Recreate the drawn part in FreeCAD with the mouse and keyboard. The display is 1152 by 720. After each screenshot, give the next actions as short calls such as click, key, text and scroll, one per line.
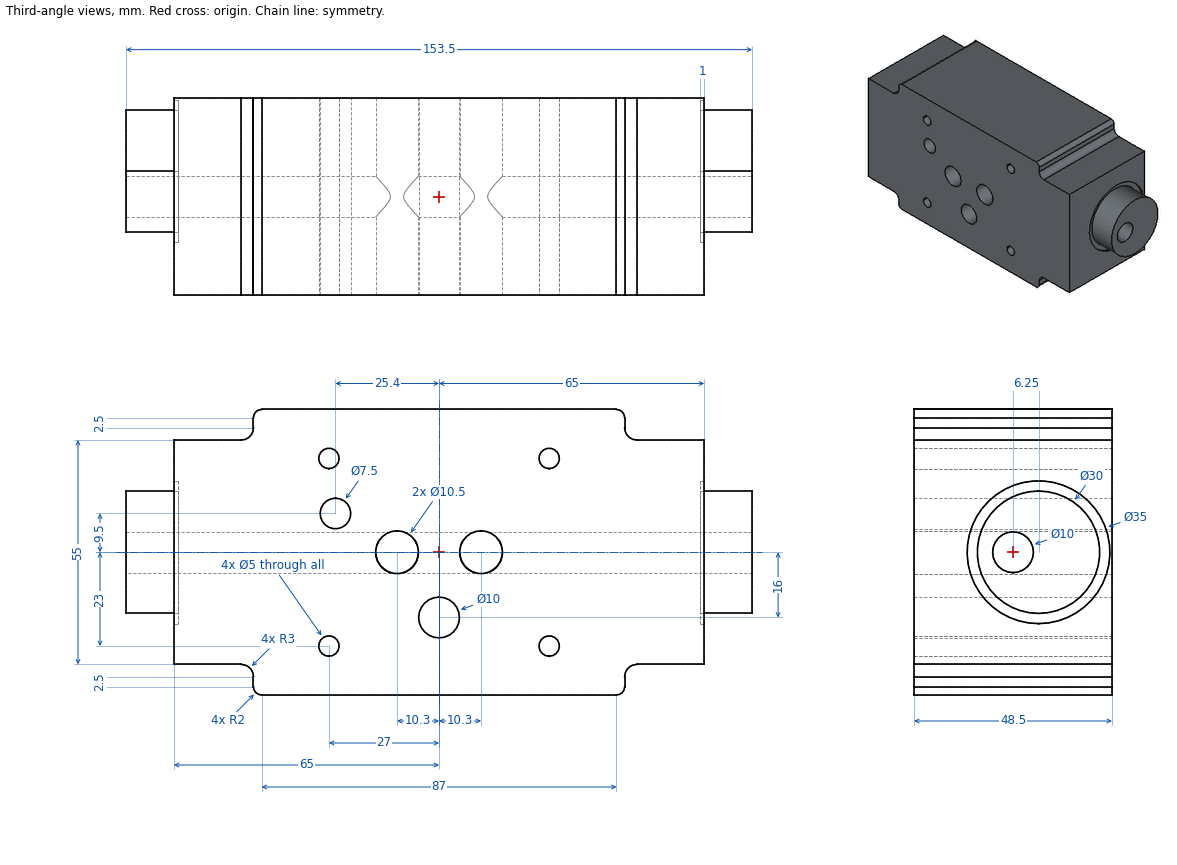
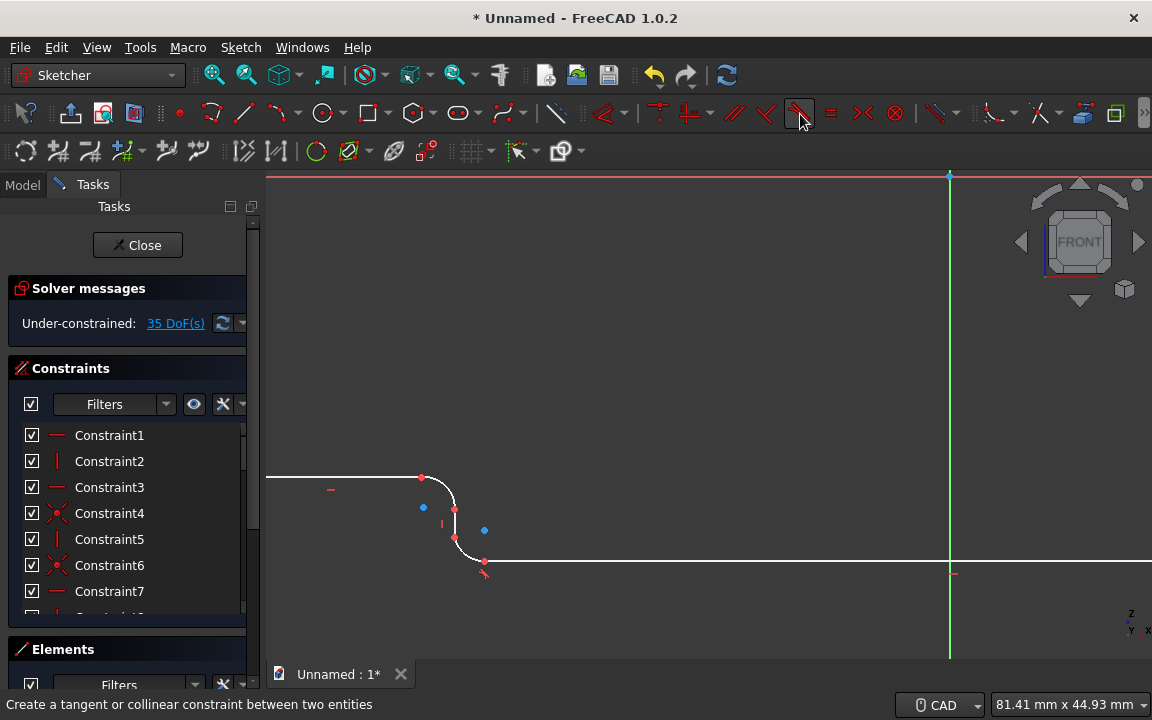
click(766, 561)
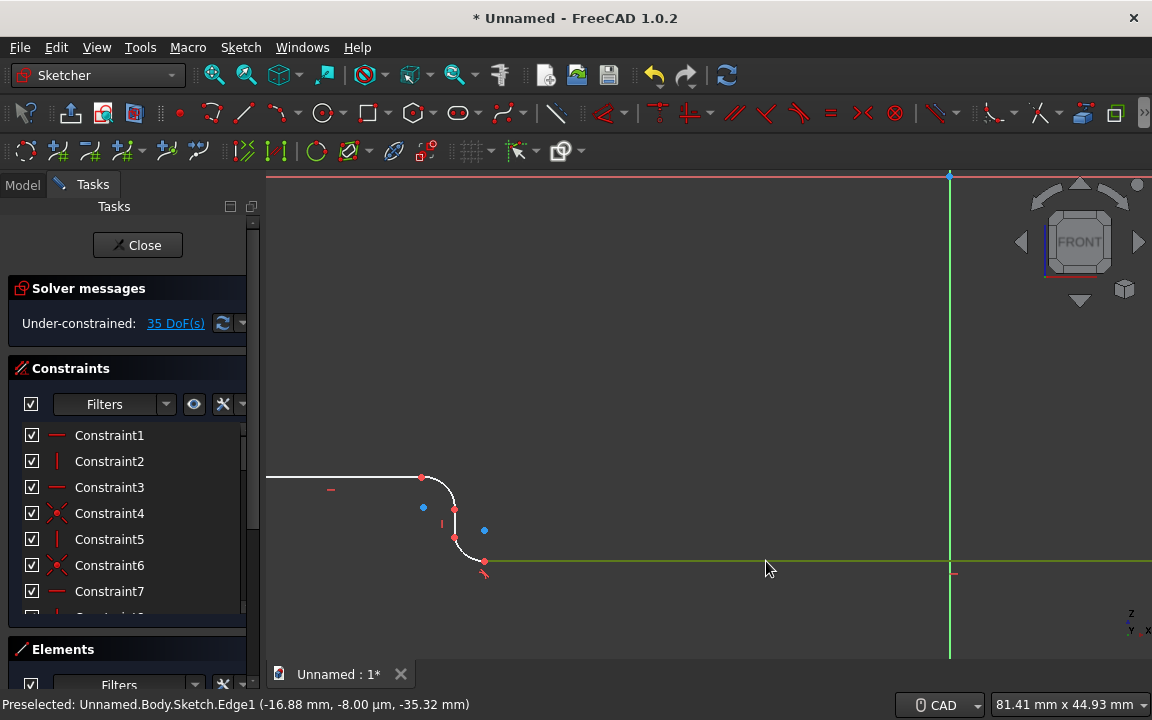
scroll(461, 553, down, 5)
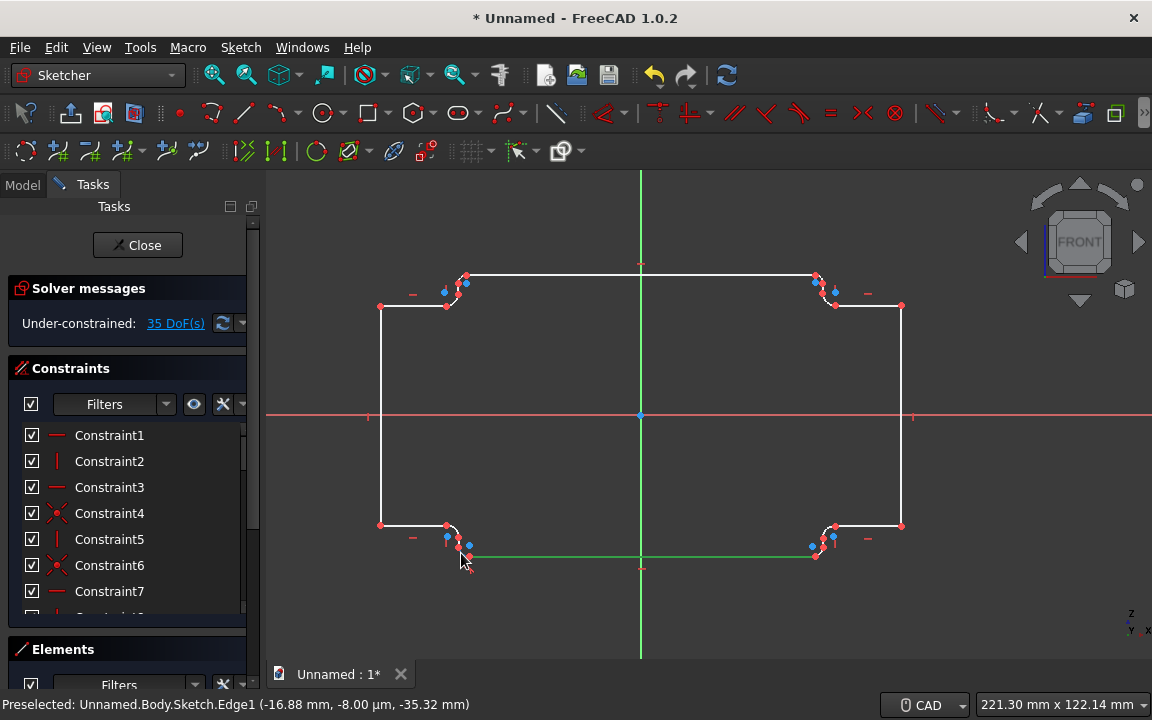
scroll(819, 555, up, 7)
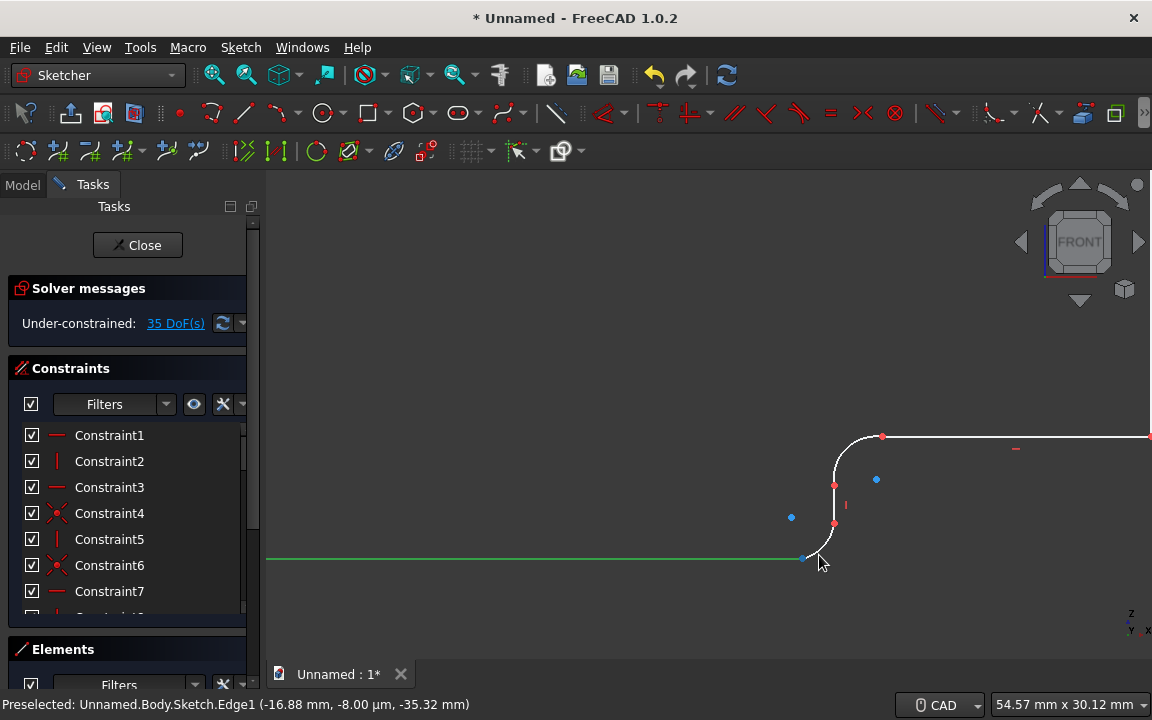
click(816, 552)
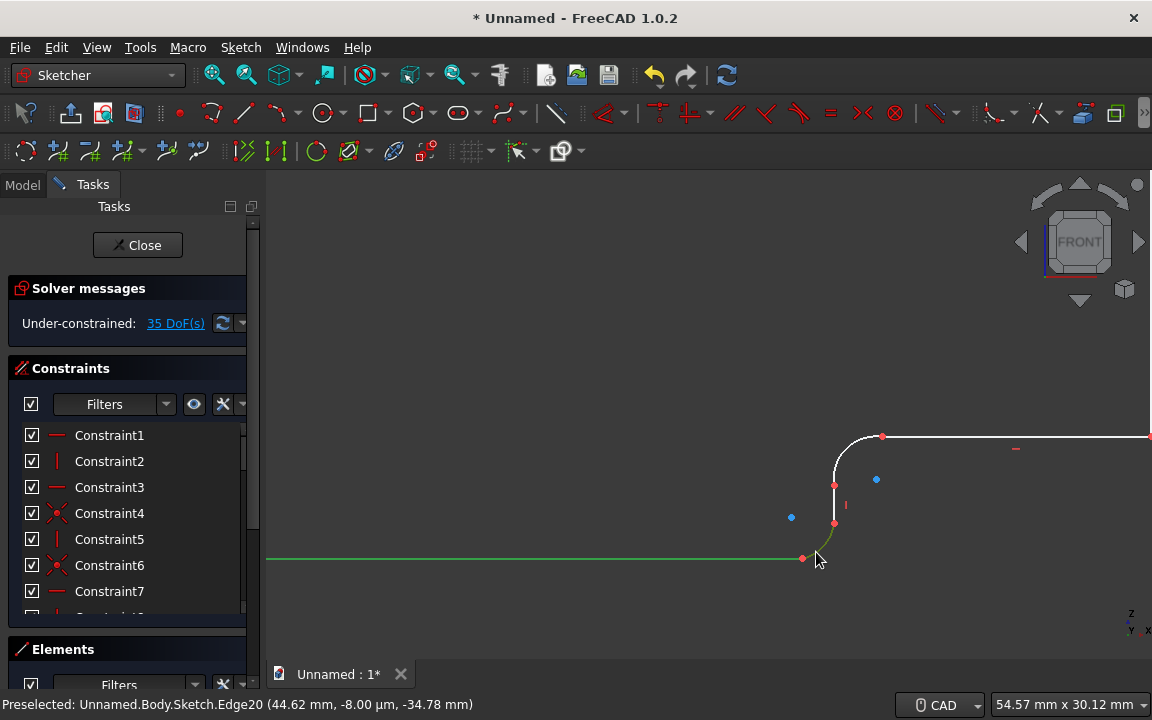
click(800, 114)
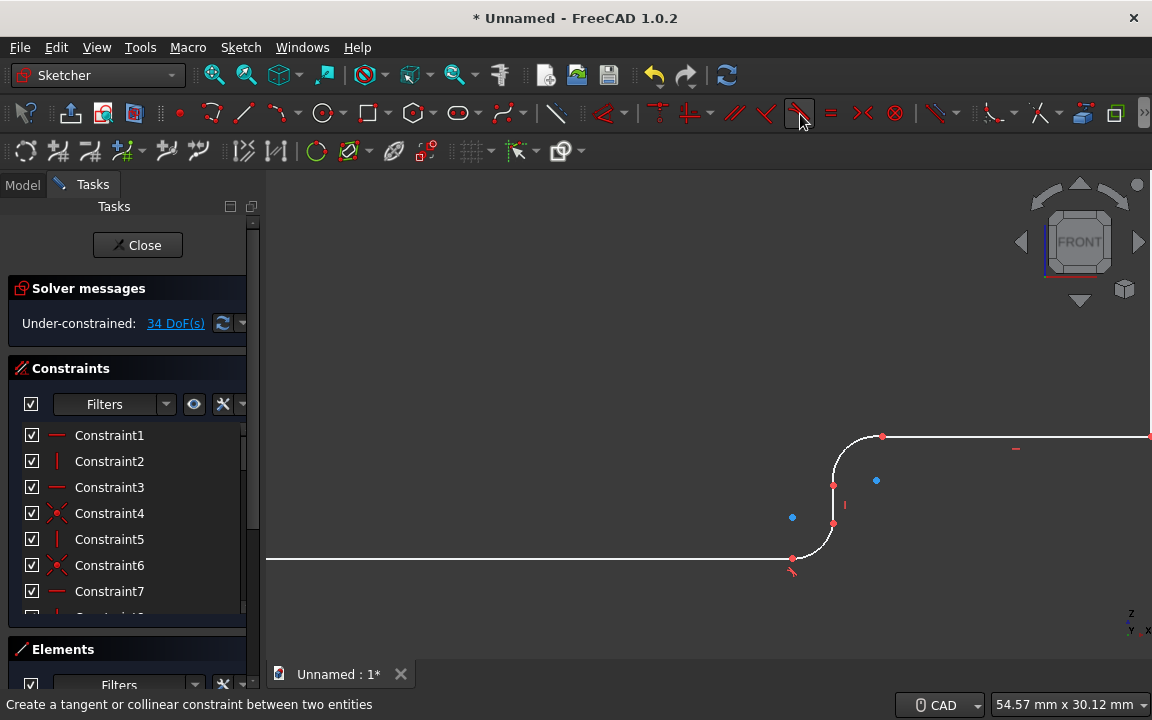
scroll(819, 555, down, 7)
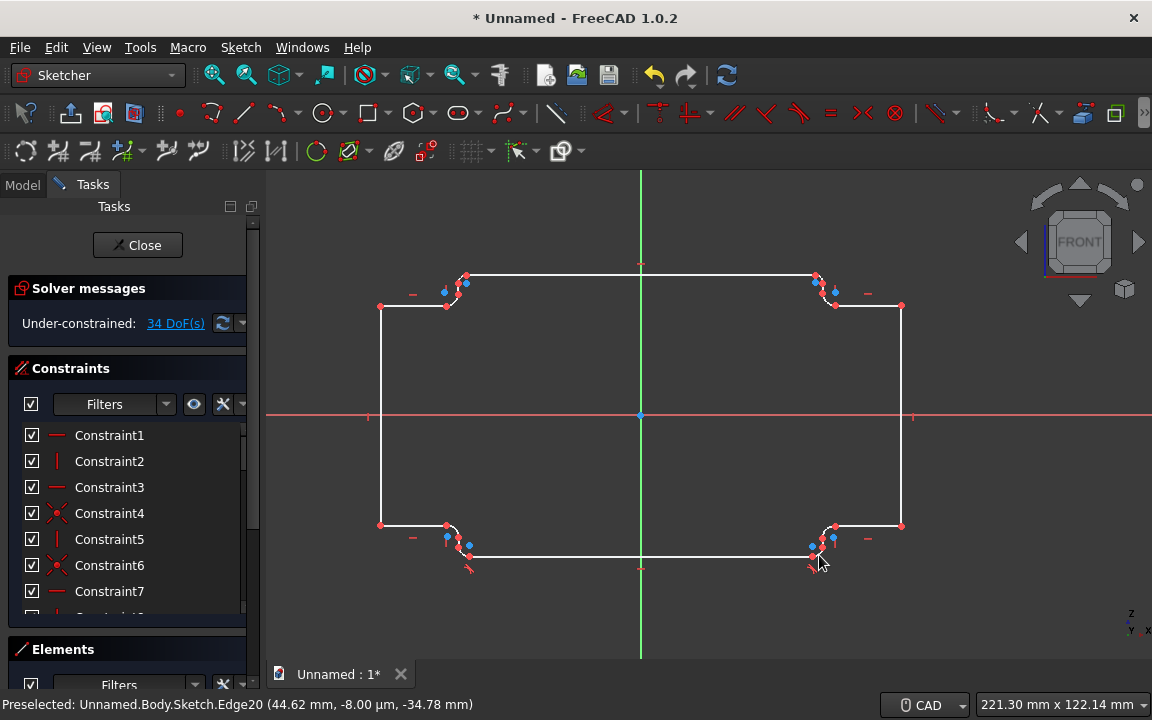
scroll(459, 545, up, 8)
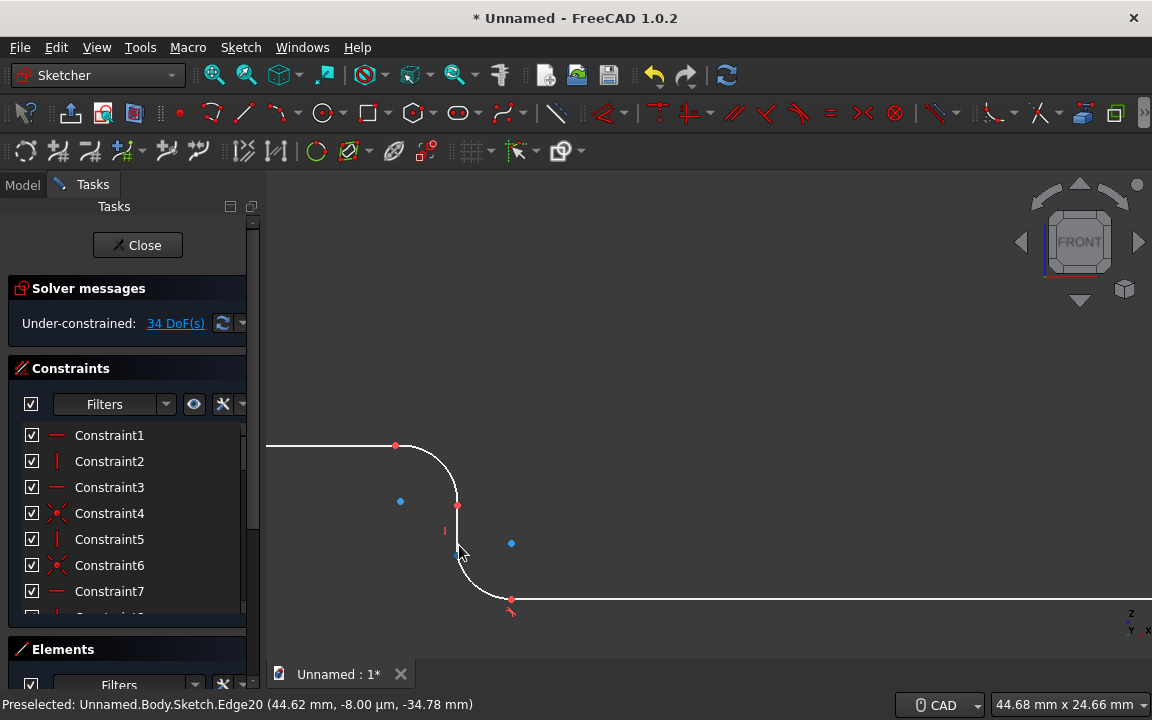
click(457, 540)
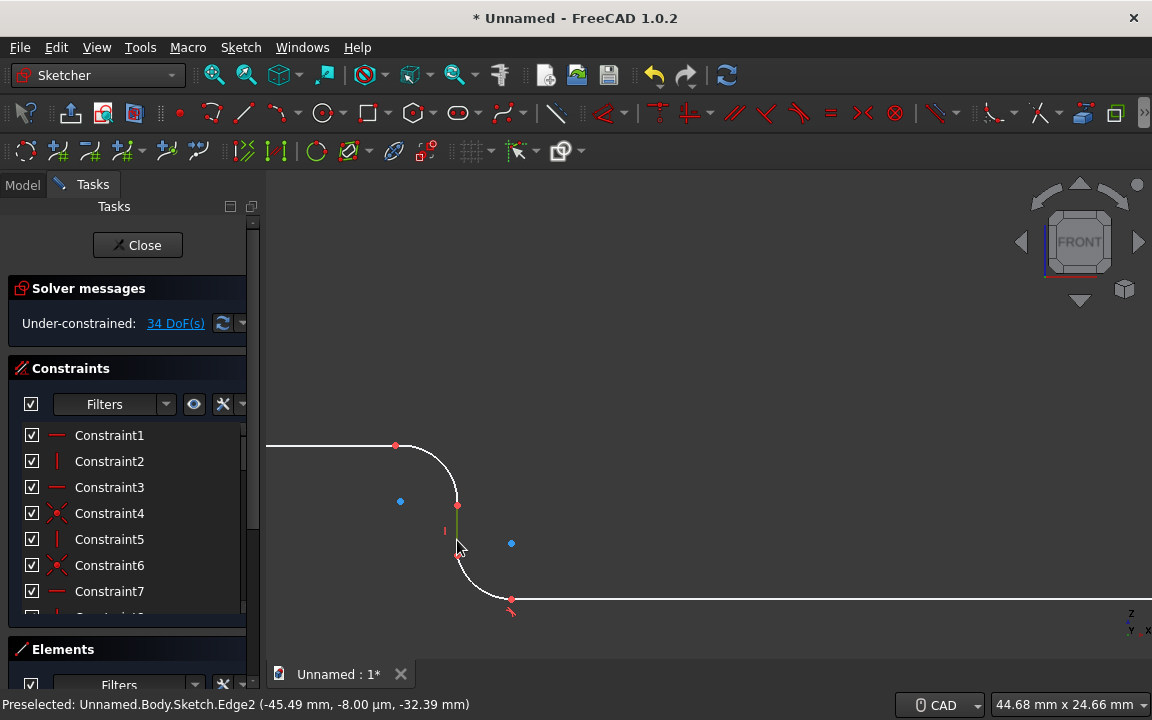
click(466, 576)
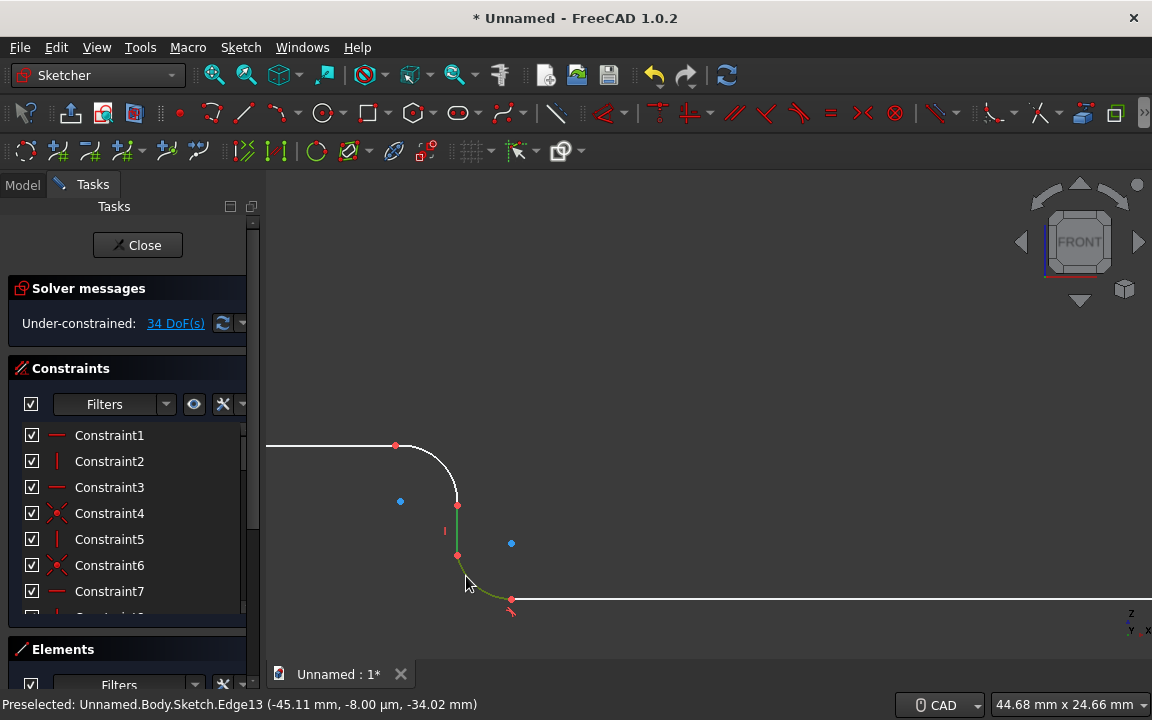
click(800, 114)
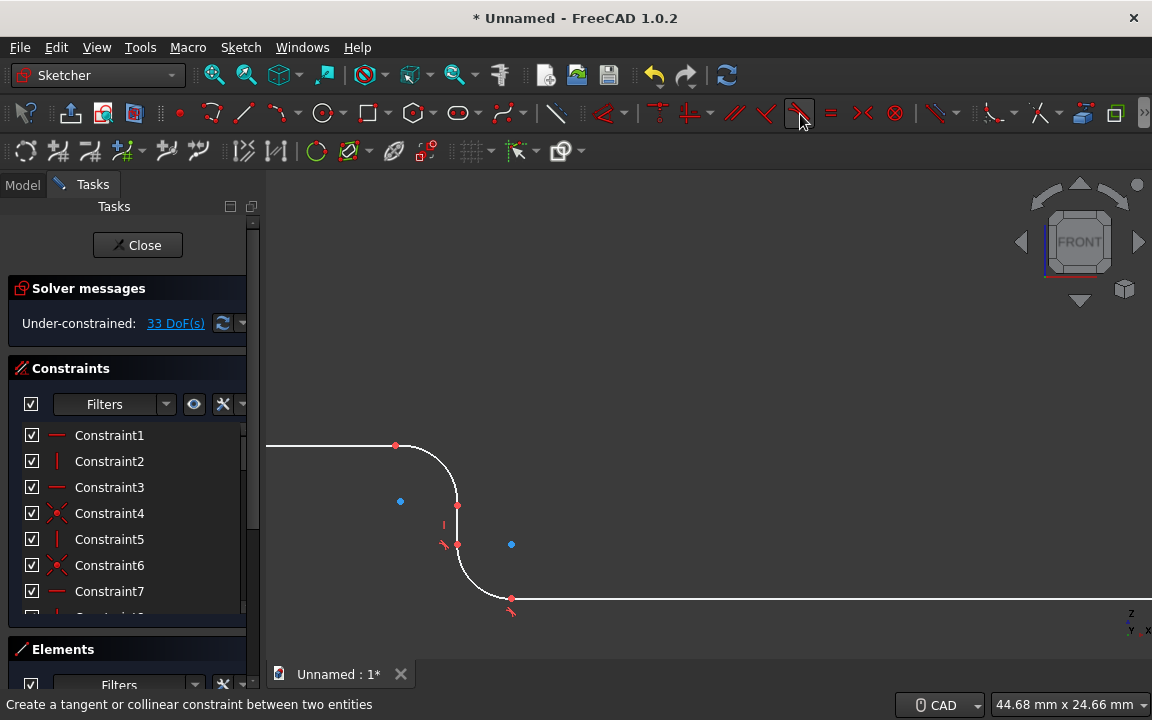
click(457, 533)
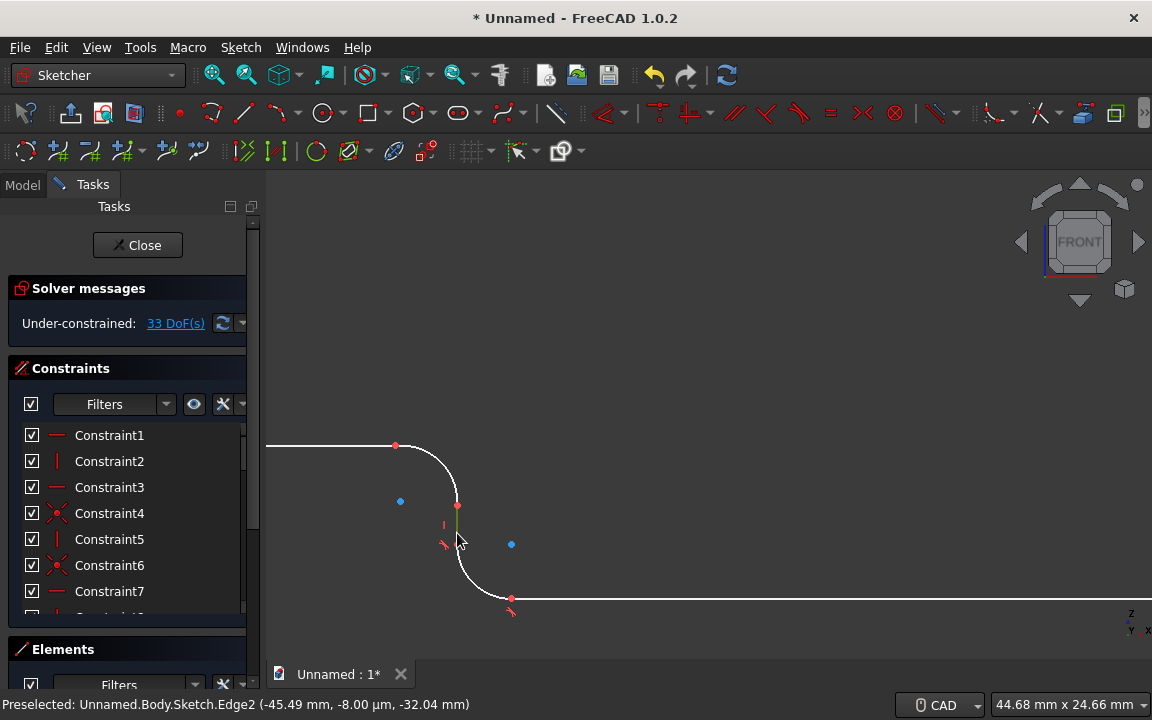
click(452, 477)